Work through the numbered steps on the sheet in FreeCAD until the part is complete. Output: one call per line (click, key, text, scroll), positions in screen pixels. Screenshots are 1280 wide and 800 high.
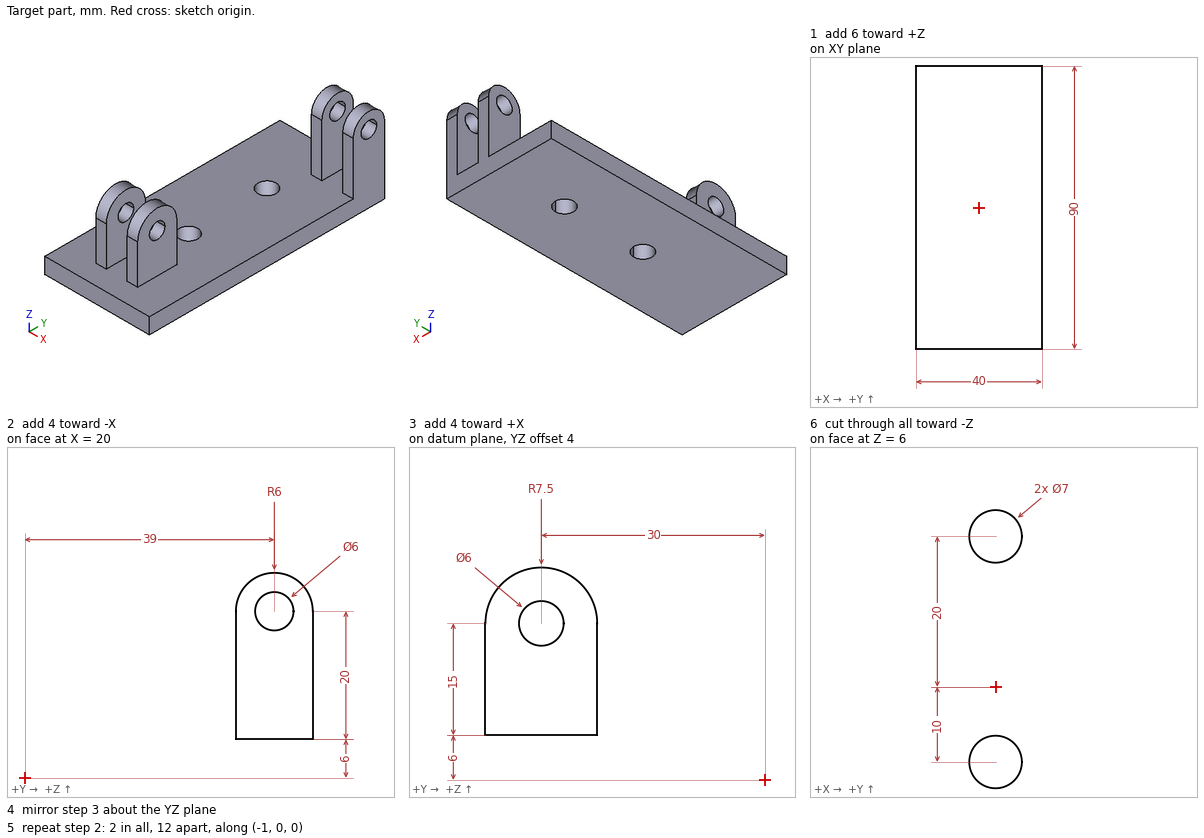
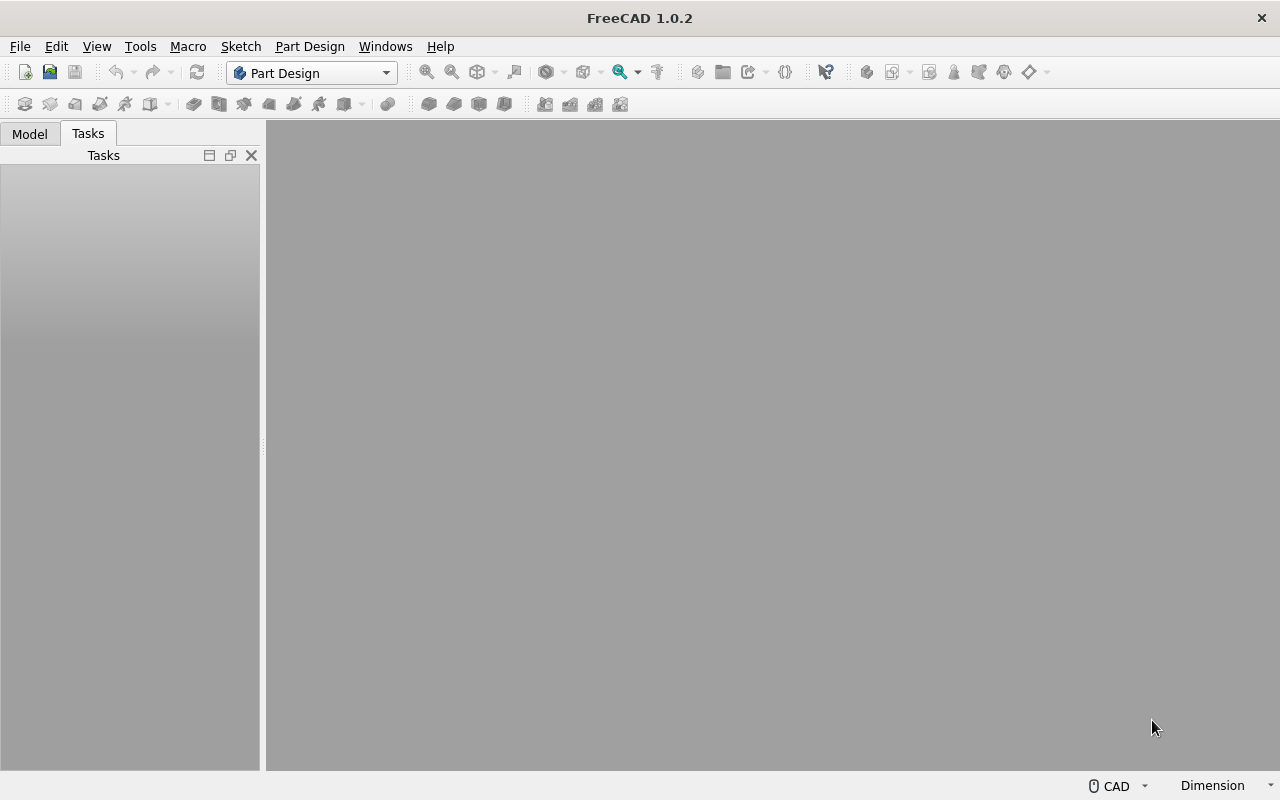
click(25, 72)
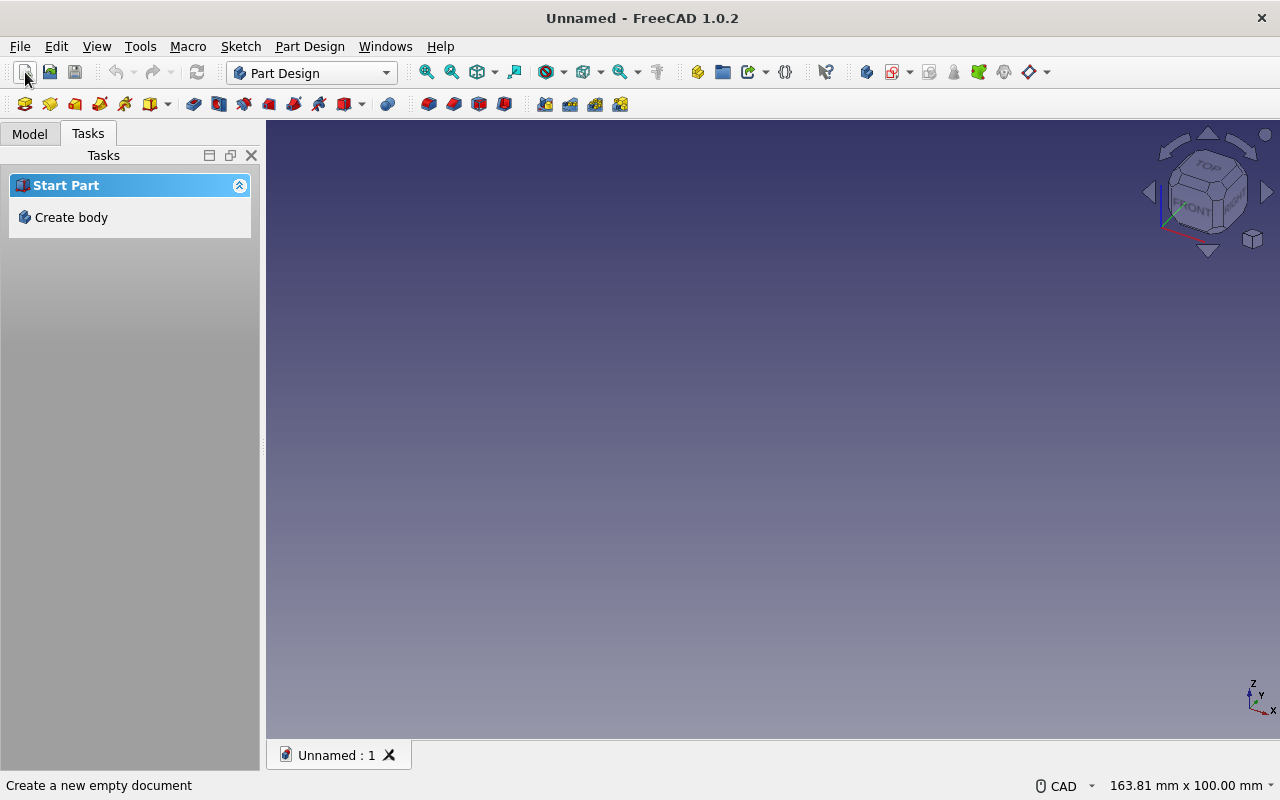
click(892, 72)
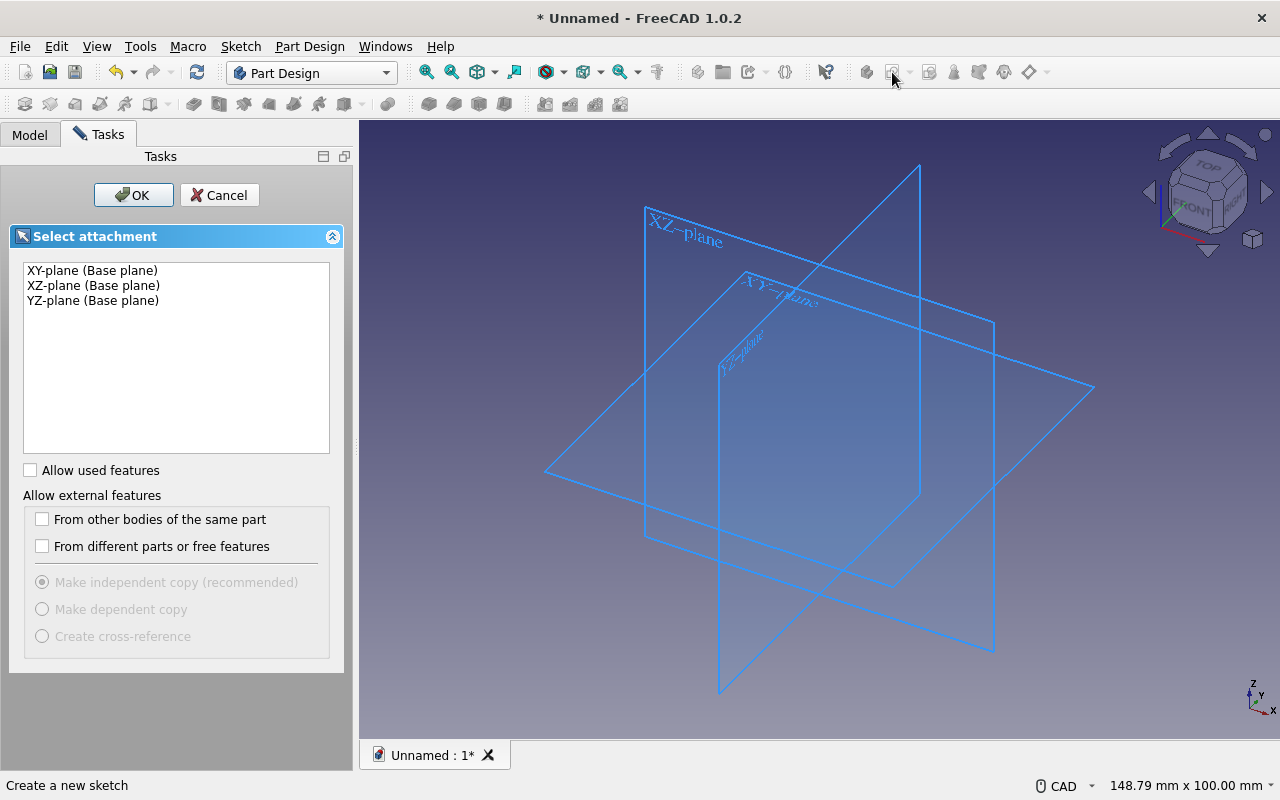
click(84, 270)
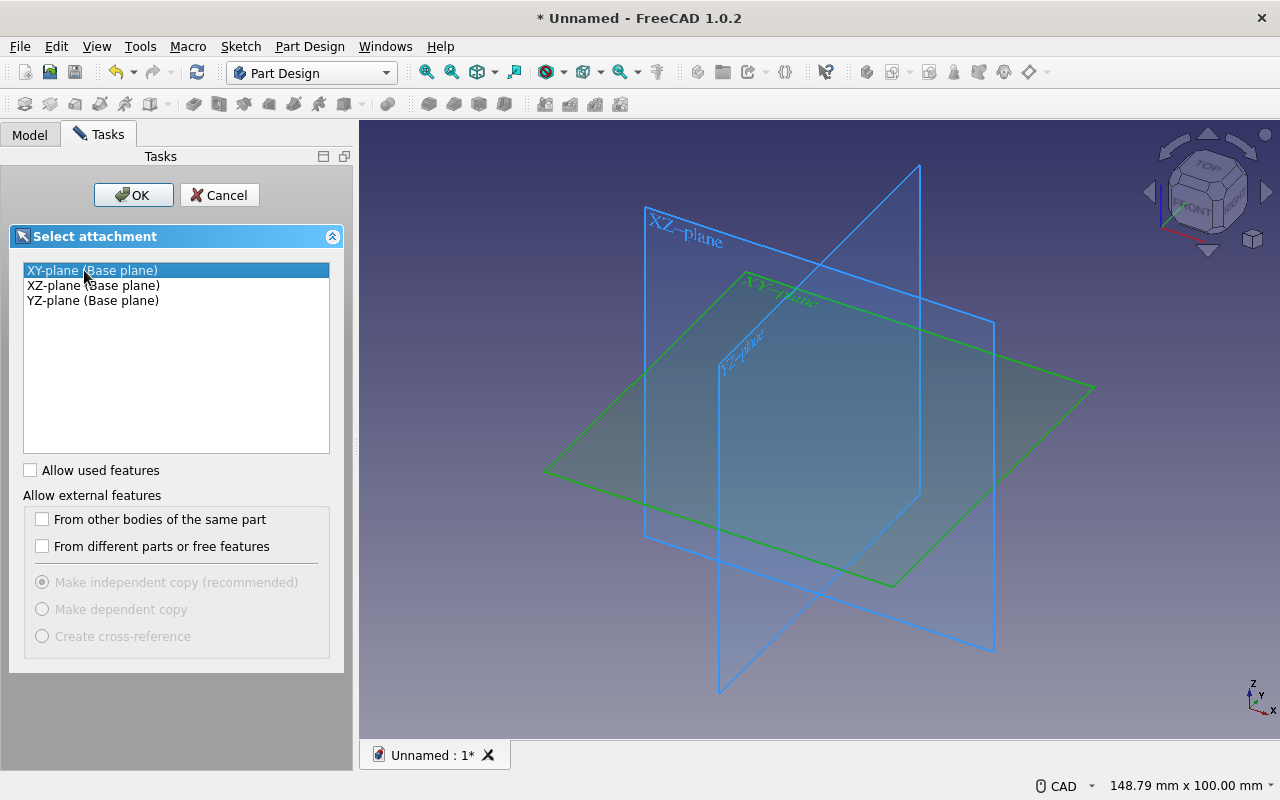
click(134, 195)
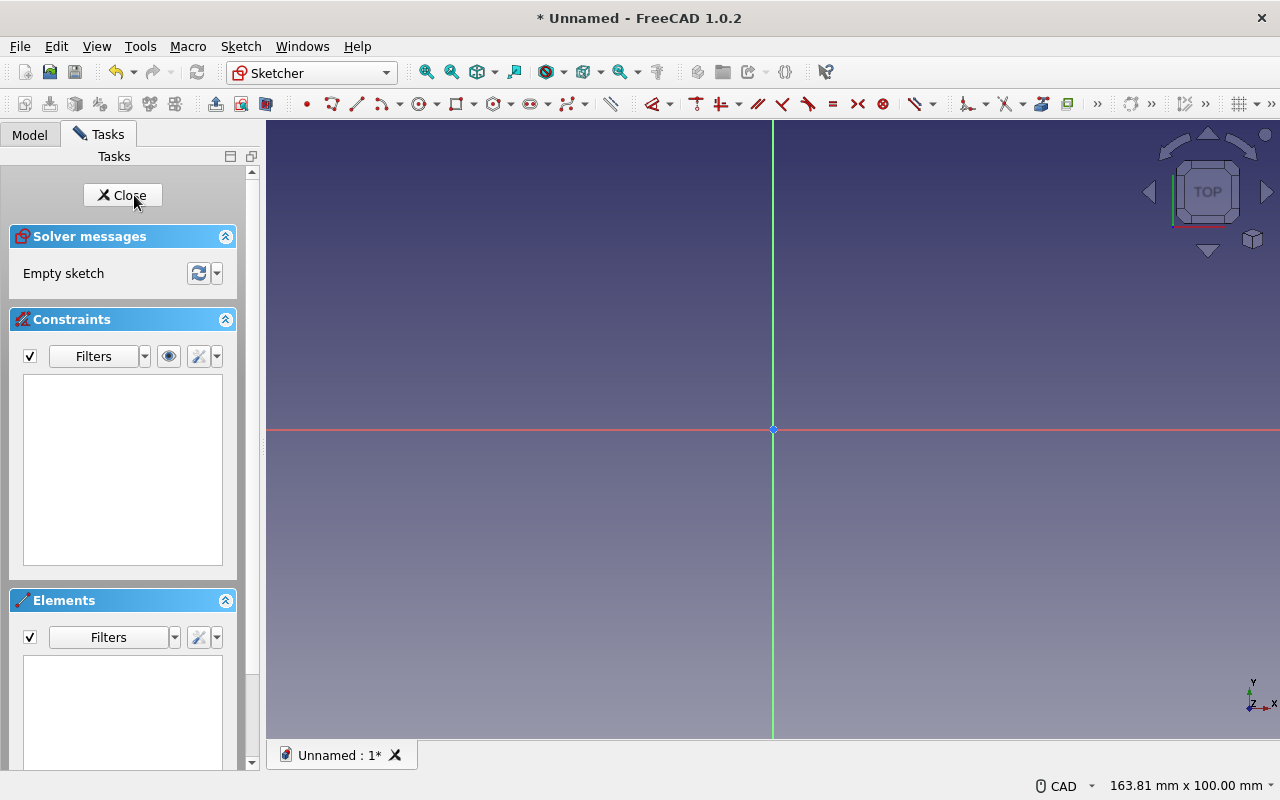
scroll(565, 429, down, 2)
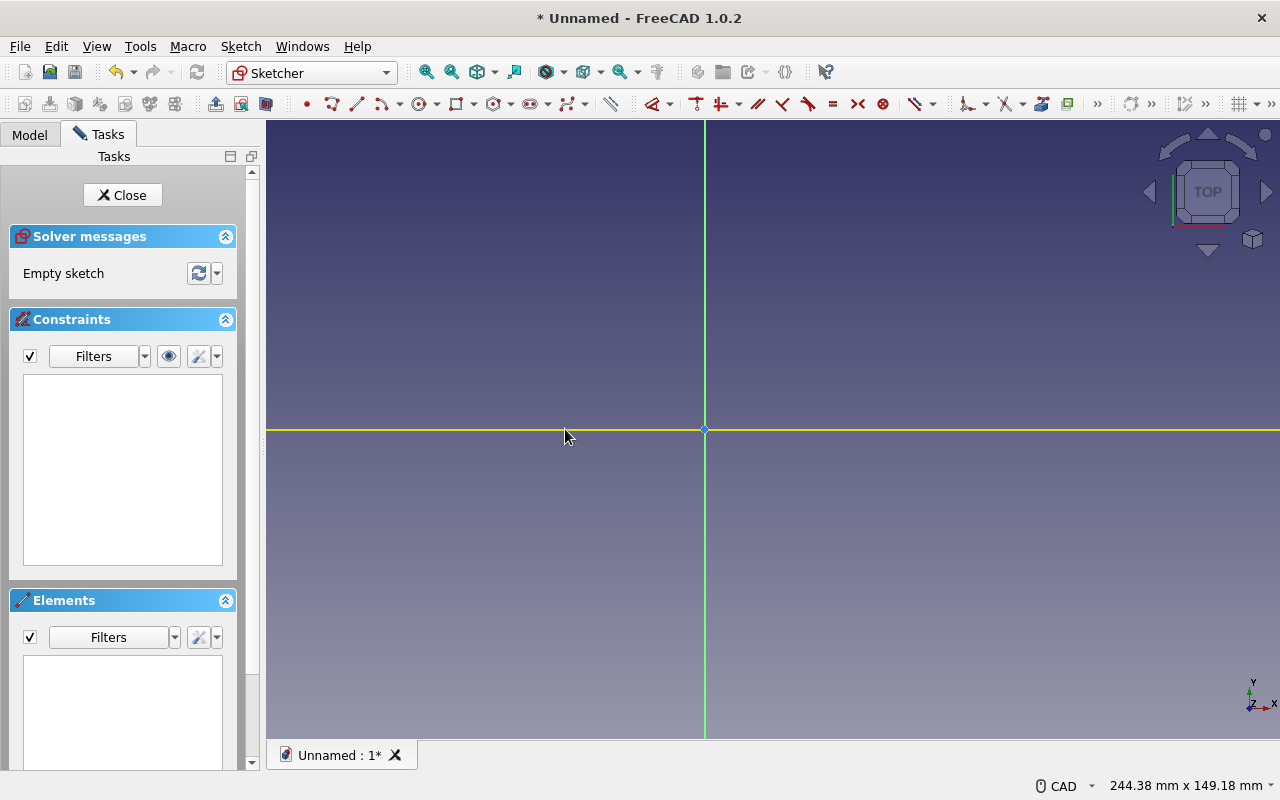
click(474, 104)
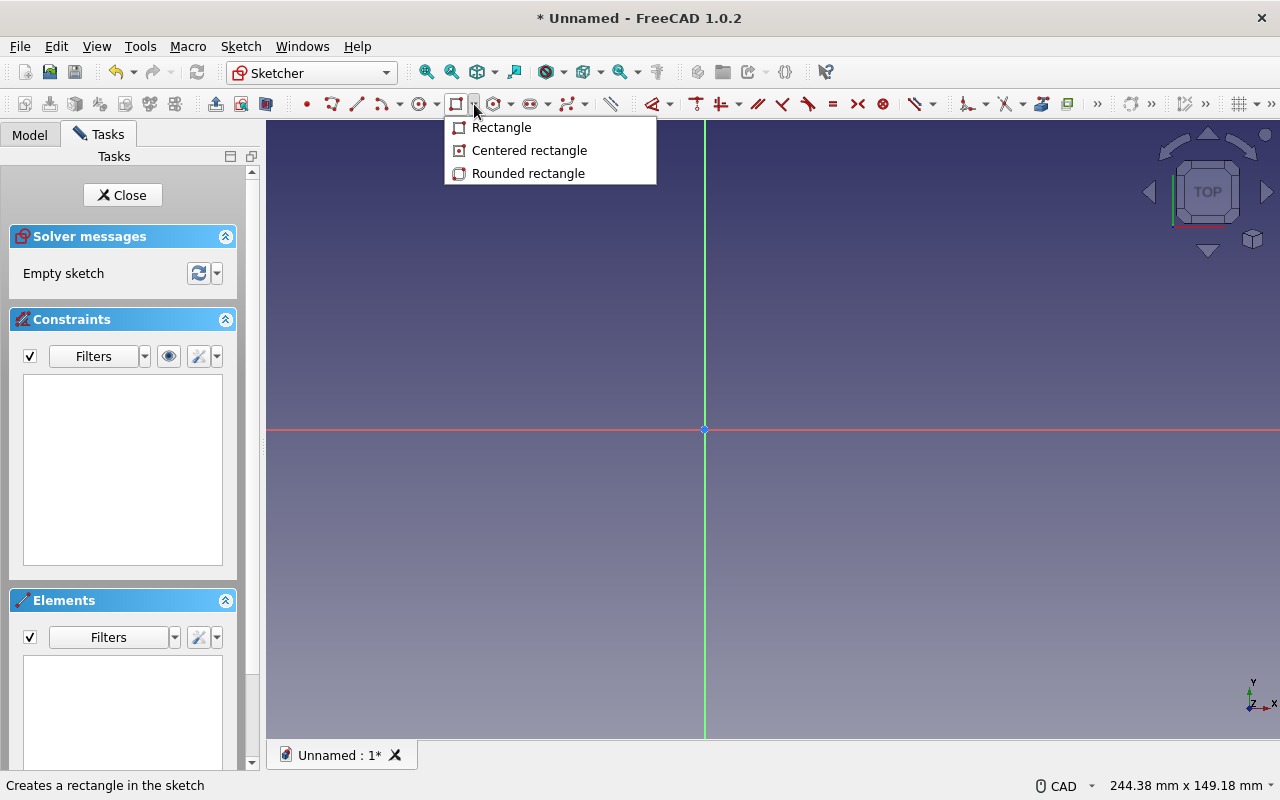
click(550, 150)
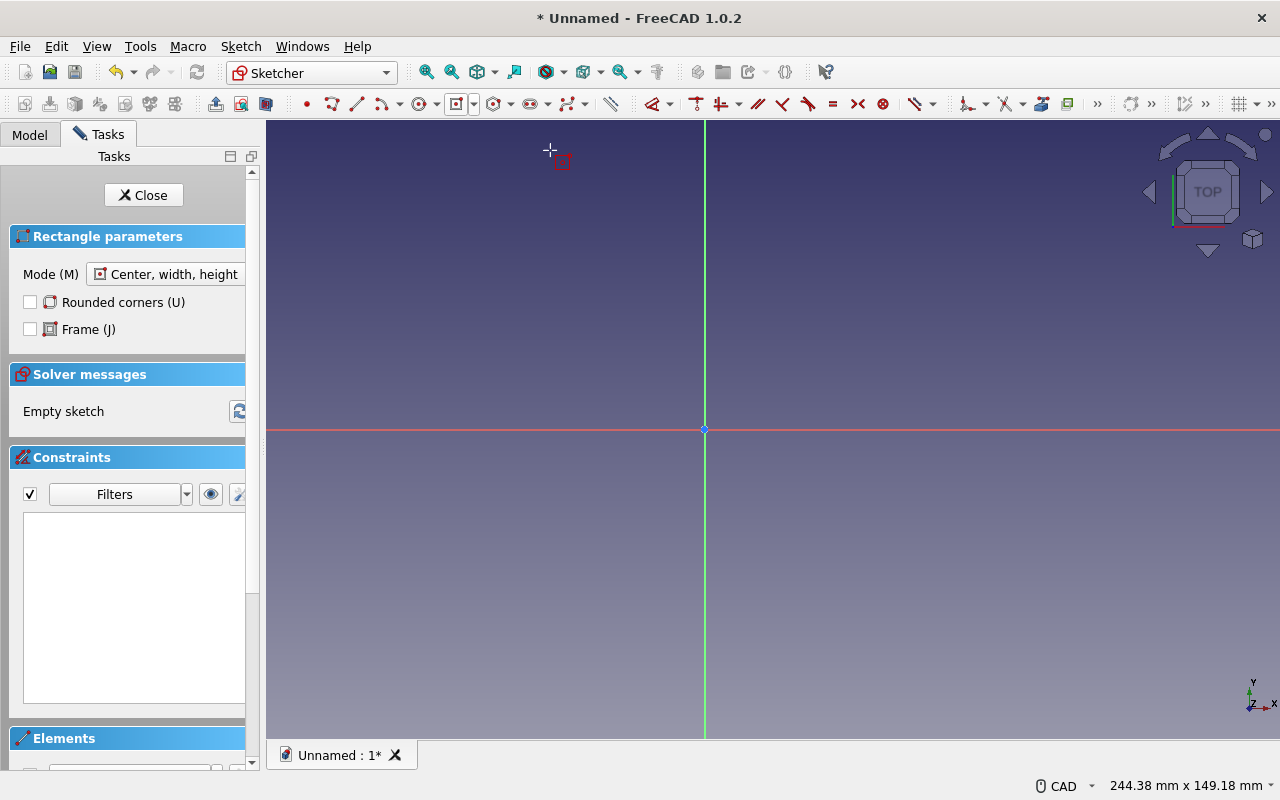
click(705, 430)
move(788, 243)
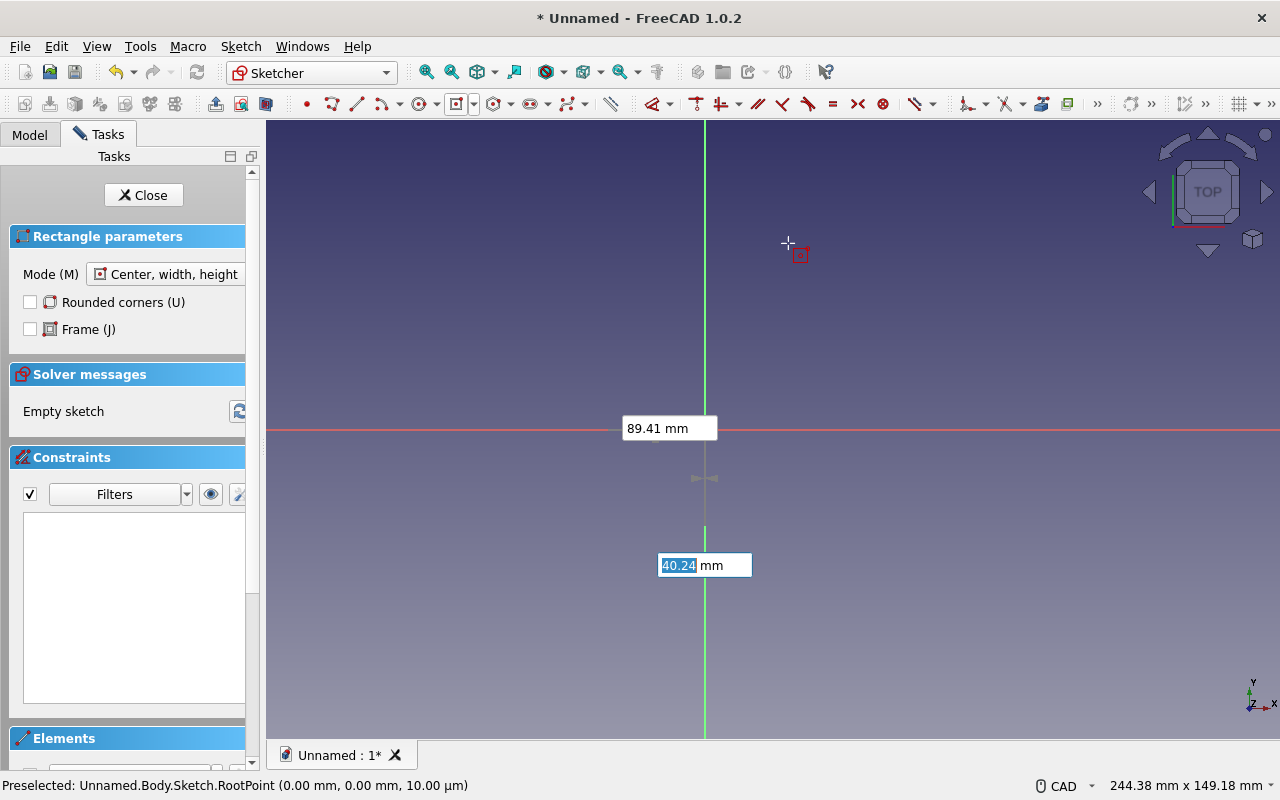
text(40)
key(Tab)
text(90)
key(Return)
key(Escape)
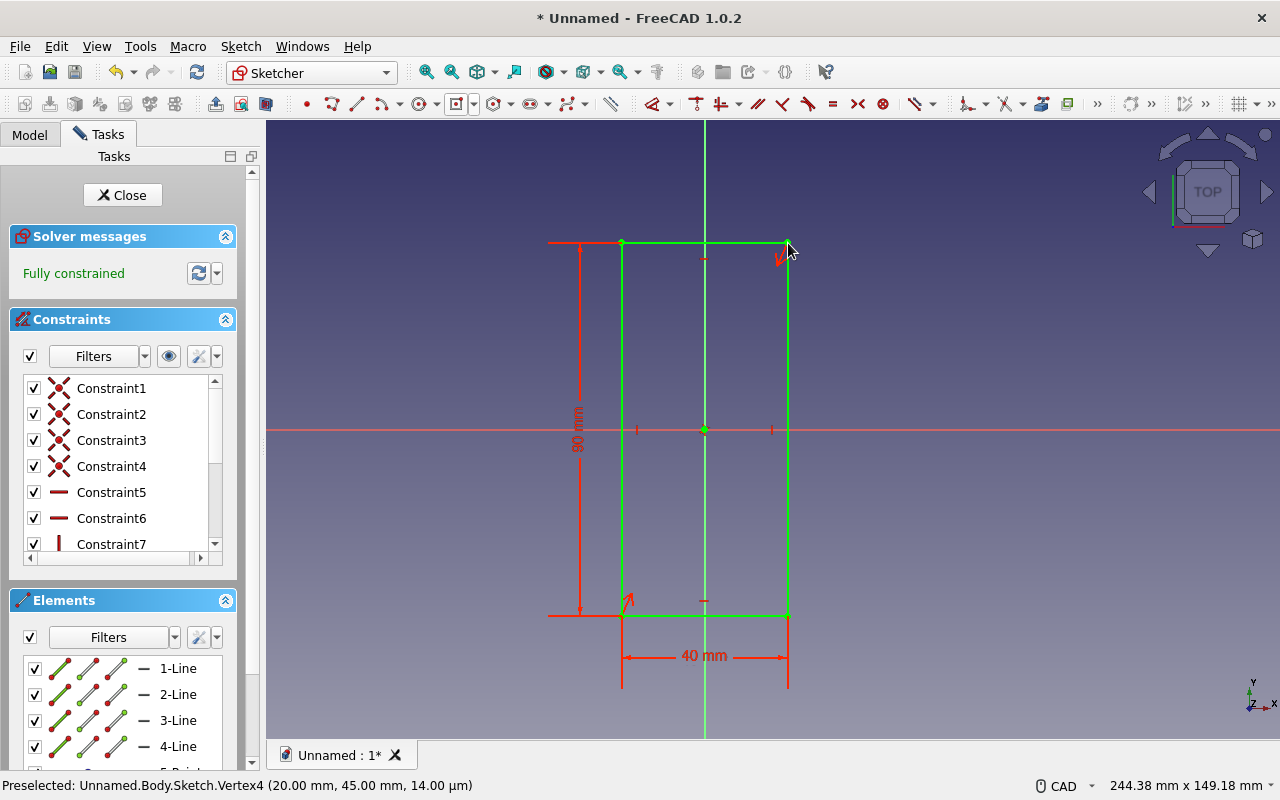
click(123, 195)